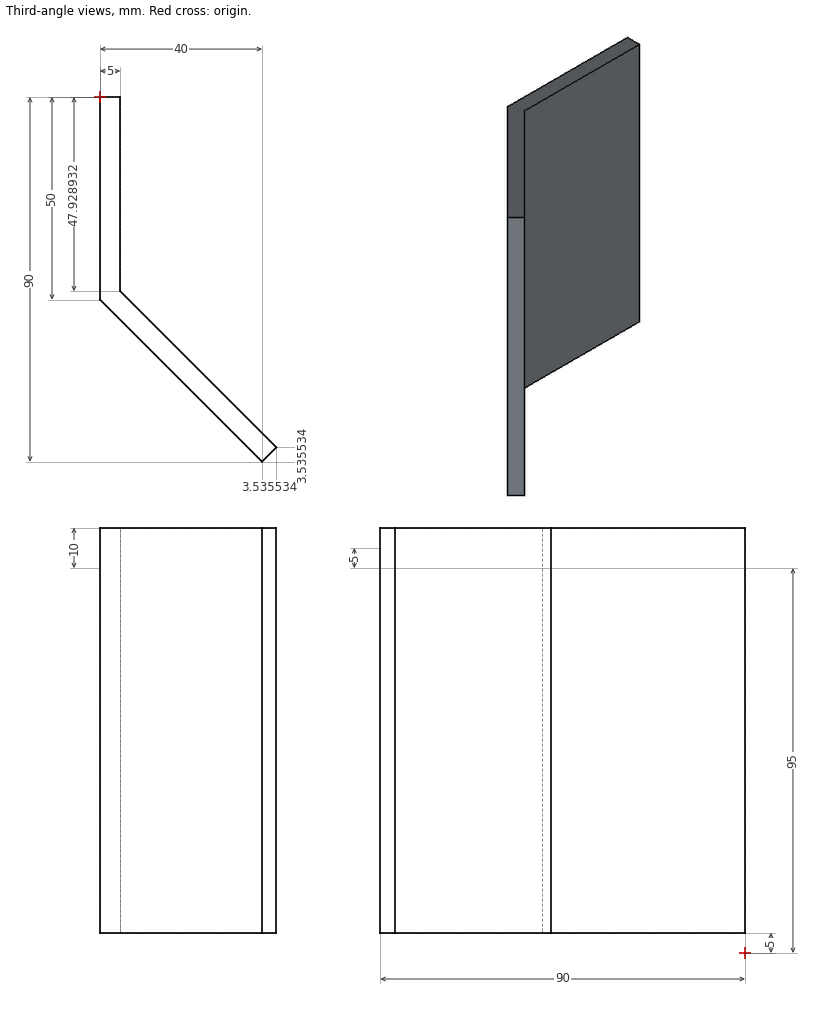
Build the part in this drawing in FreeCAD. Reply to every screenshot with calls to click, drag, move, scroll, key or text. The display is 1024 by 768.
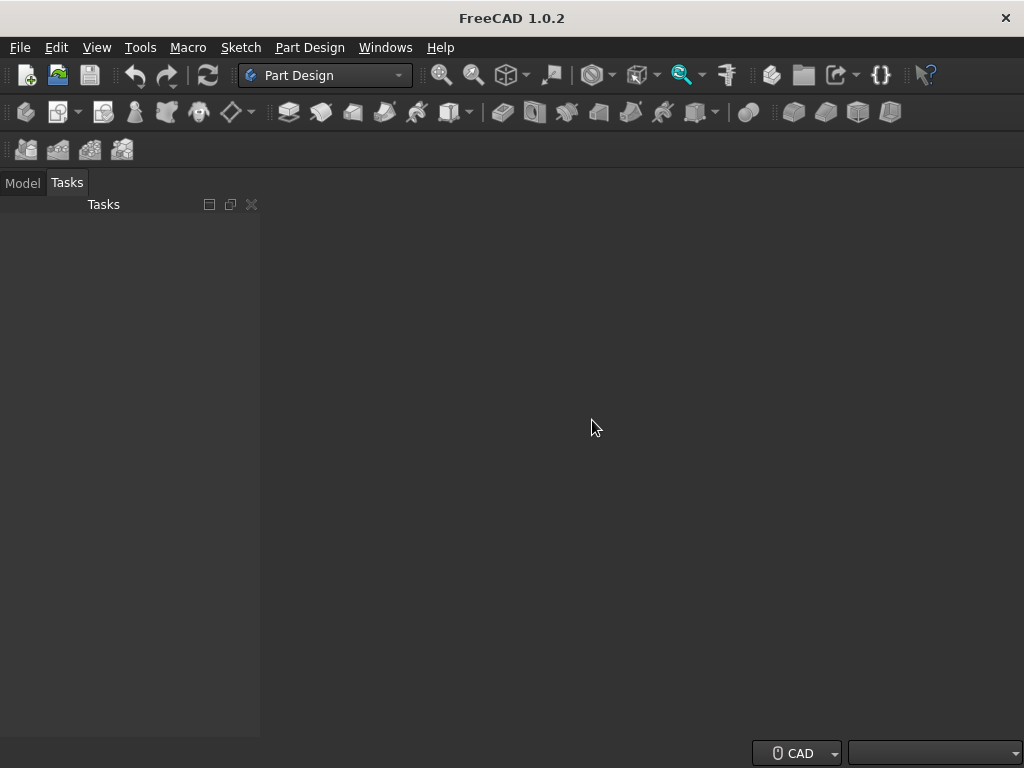
click(26, 76)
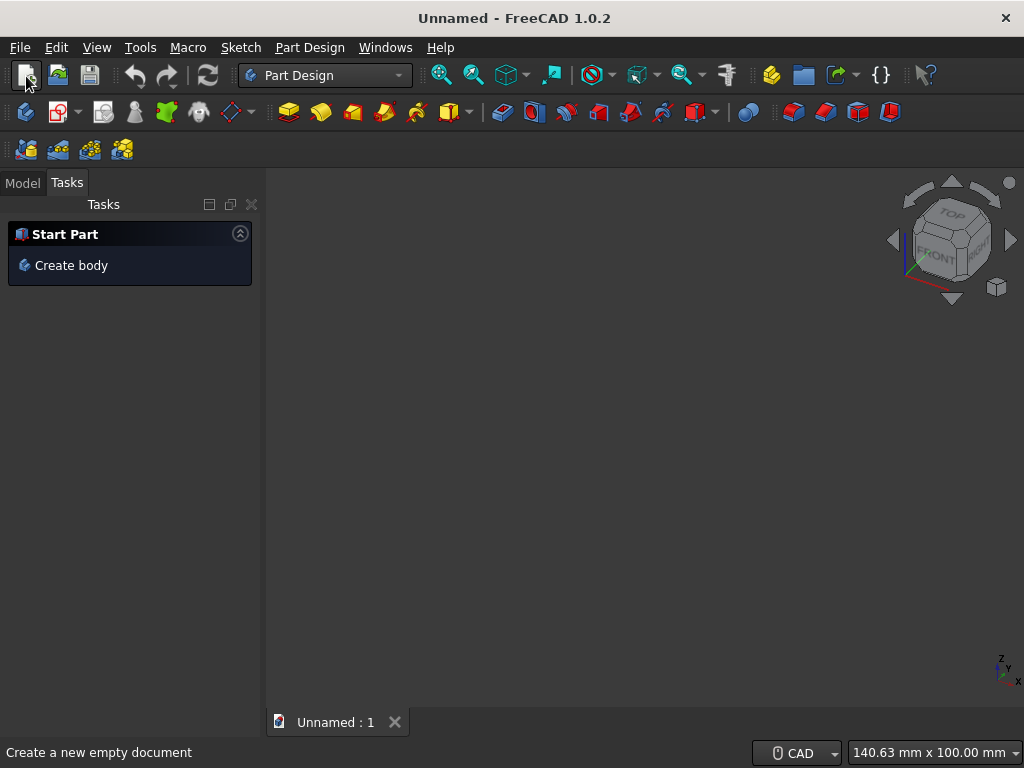
click(58, 112)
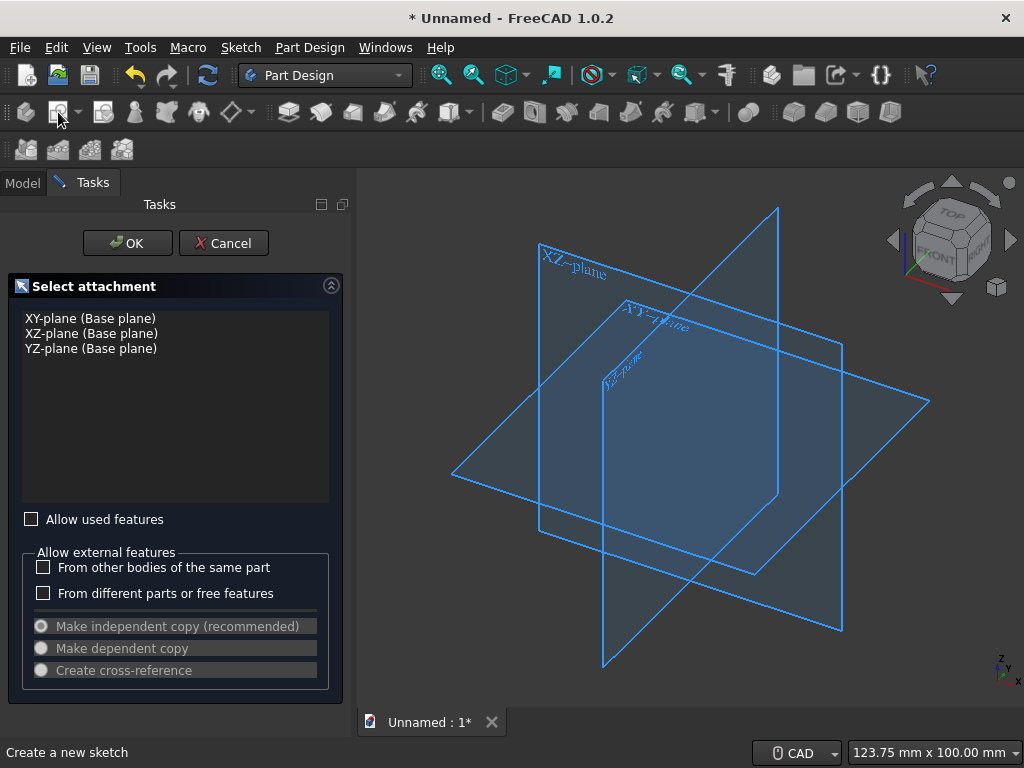
click(82, 318)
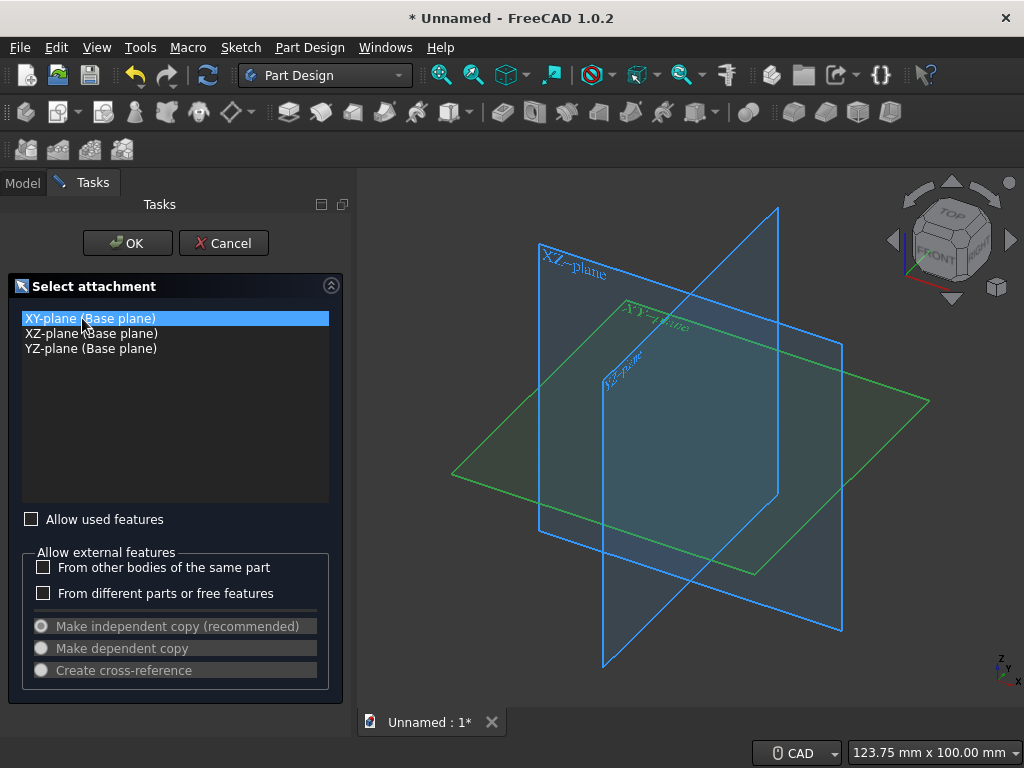
click(128, 243)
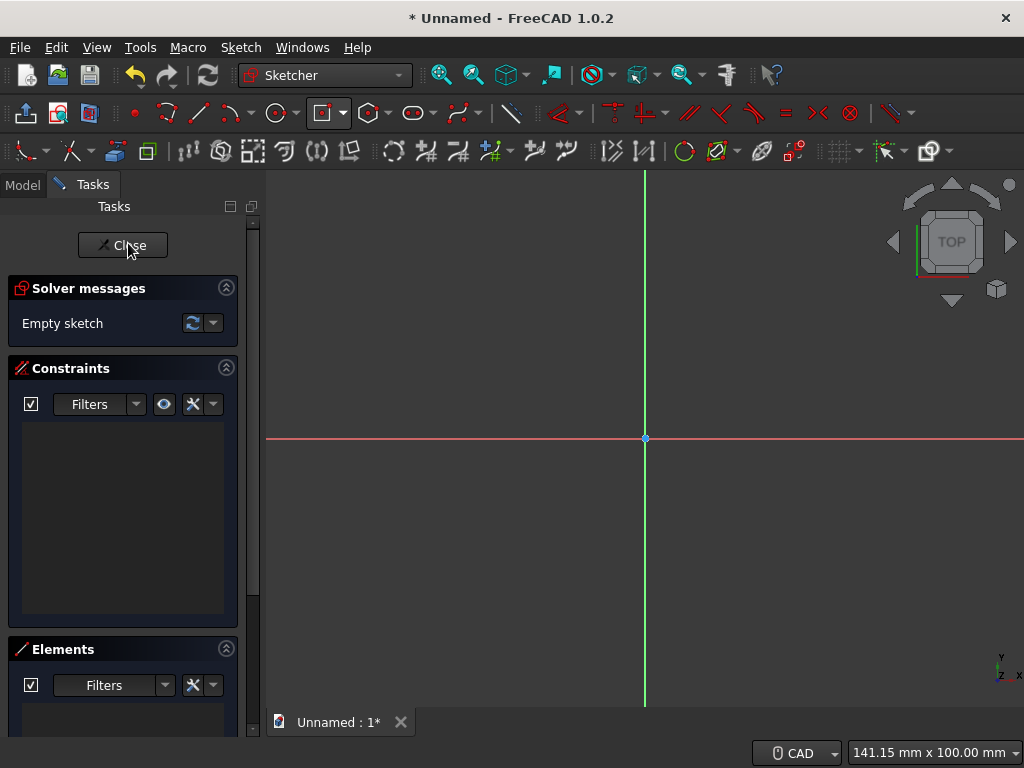
scroll(351, 198, down, 3)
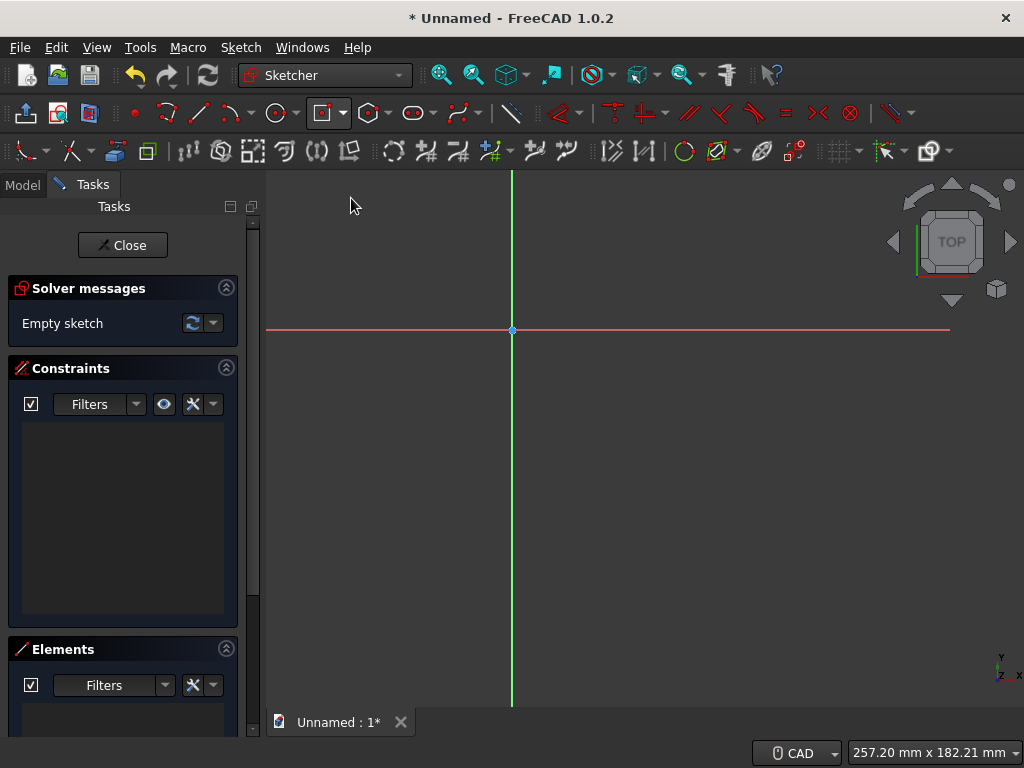
click(168, 114)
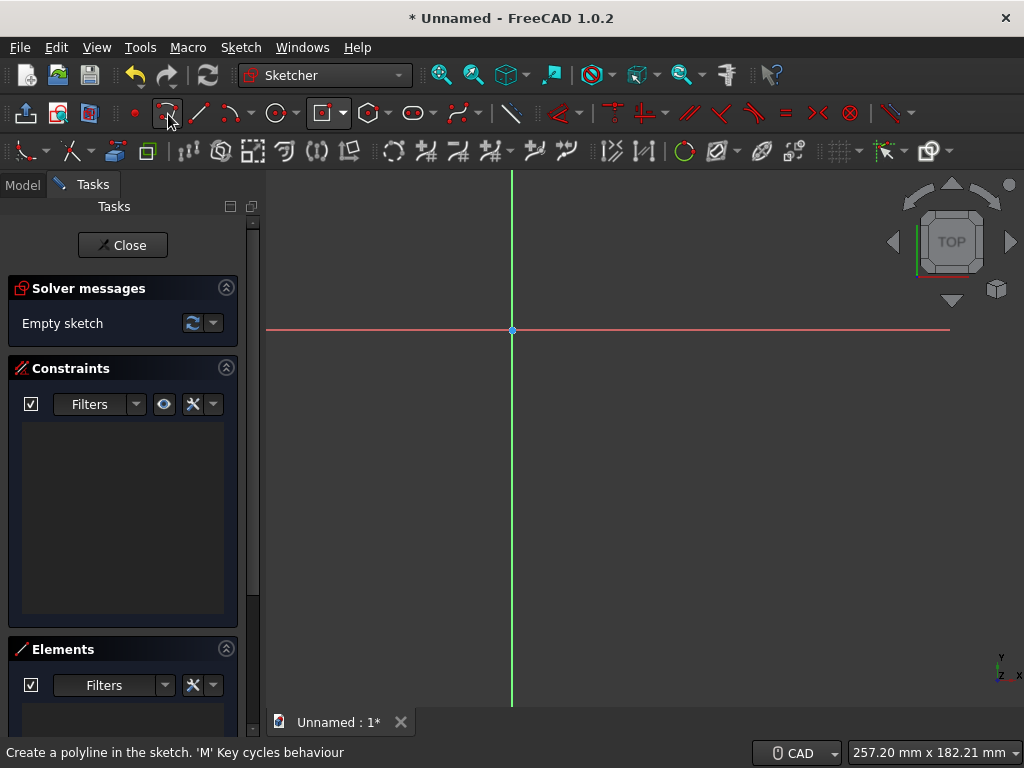
click(512, 330)
click(521, 477)
click(630, 595)
click(641, 585)
click(527, 471)
click(527, 339)
click(512, 330)
key(Escape)
key(Escape)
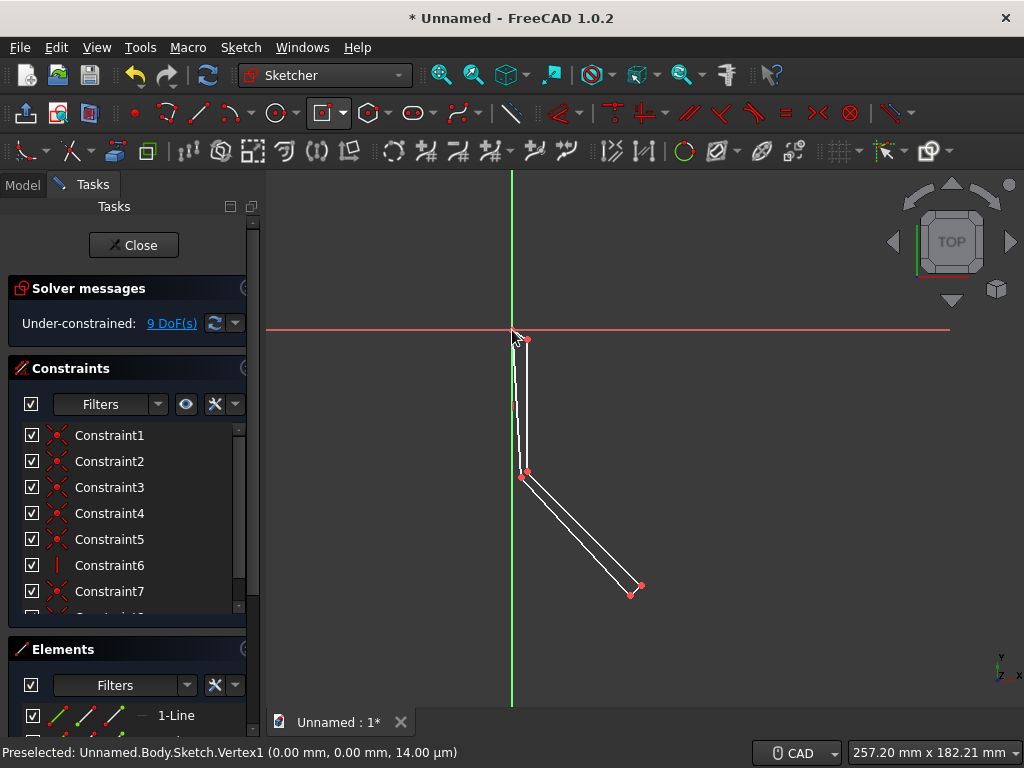
click(515, 374)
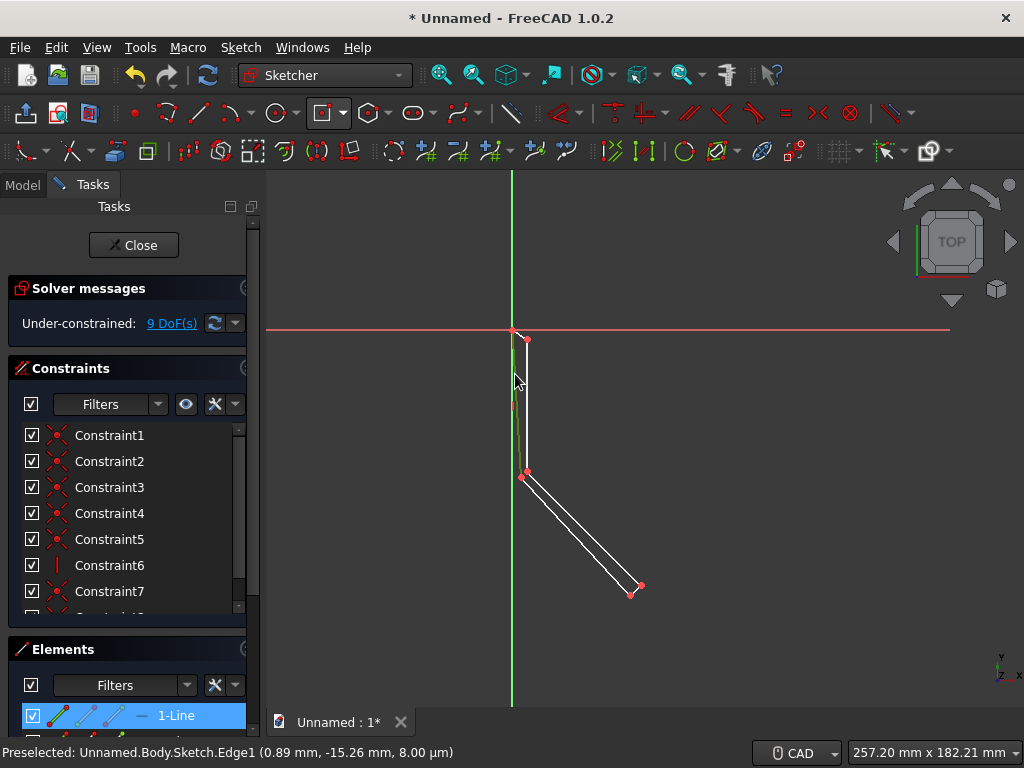
key(v)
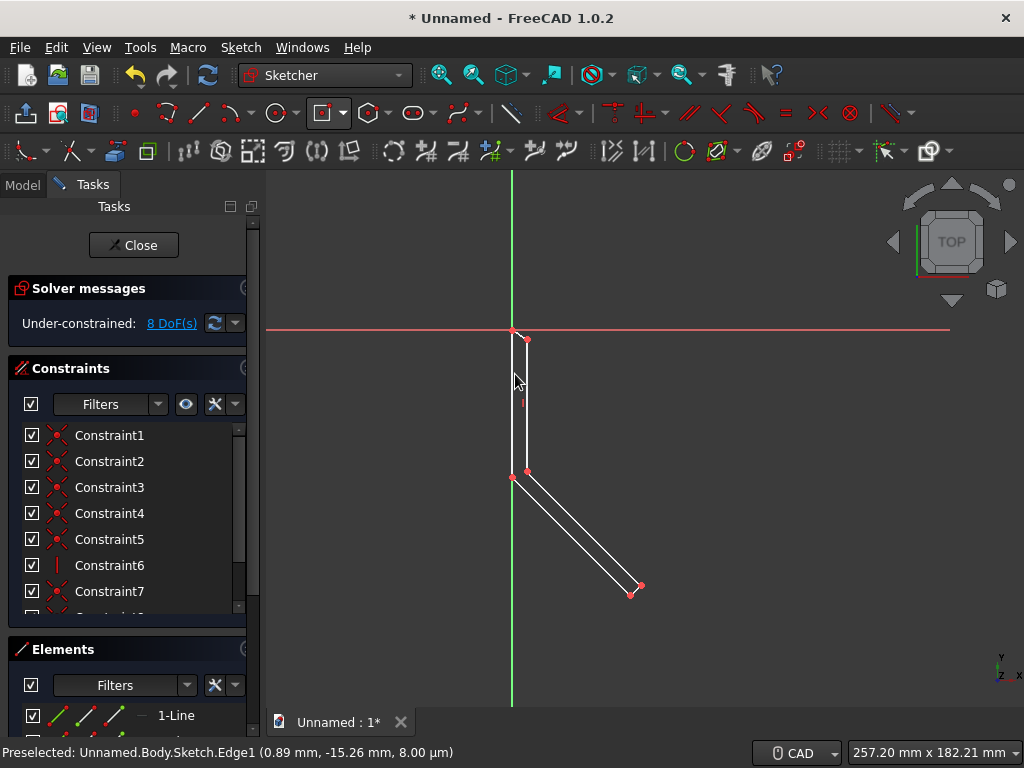
scroll(521, 336, up, 5)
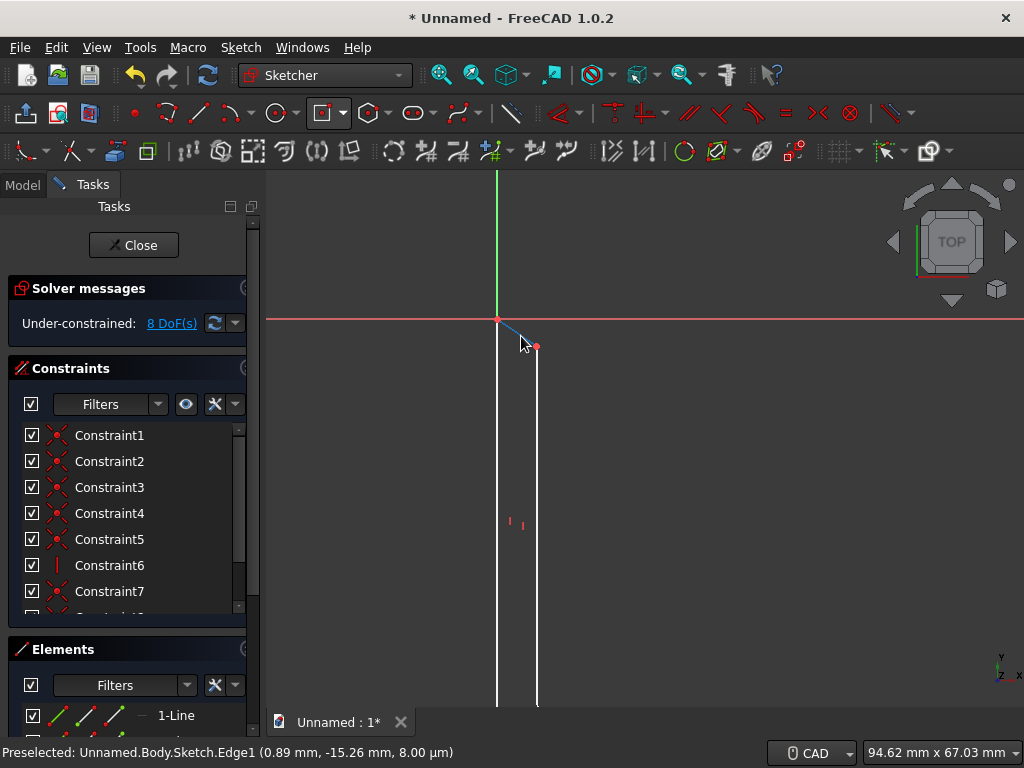
click(521, 335)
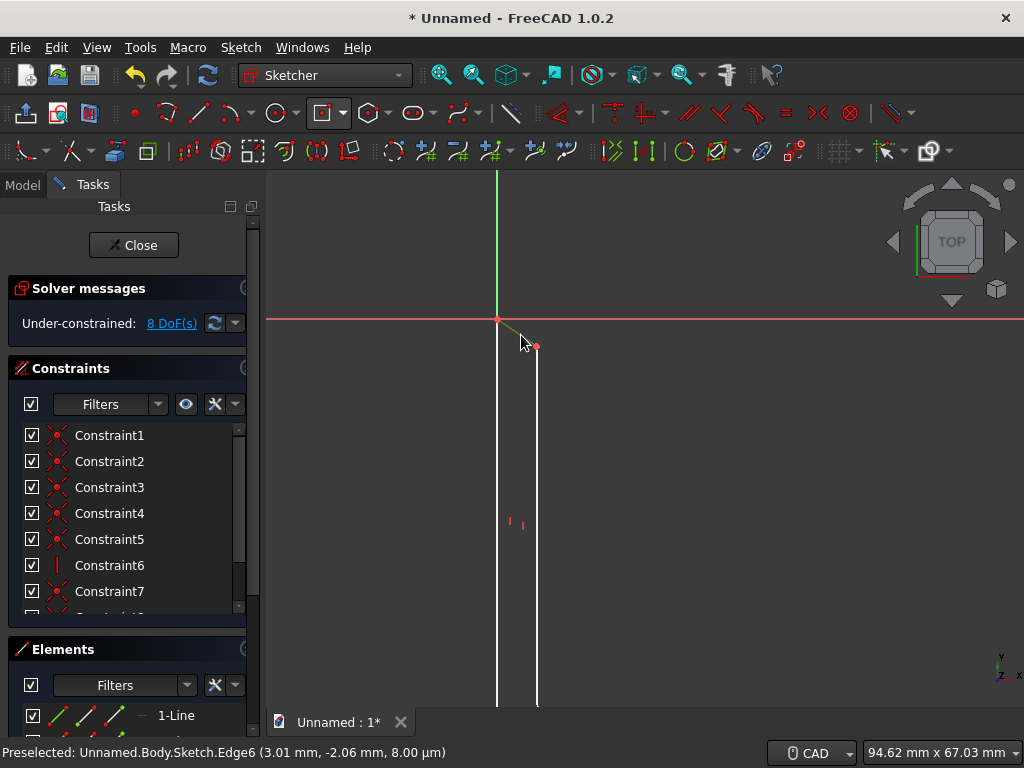
key(h)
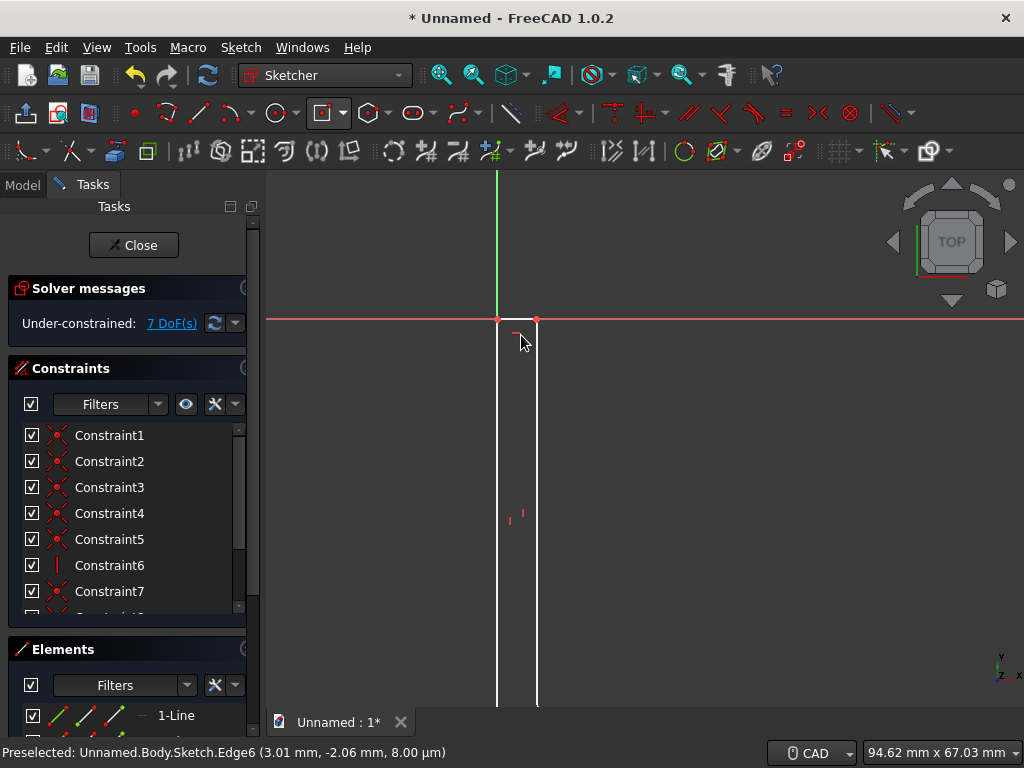
click(558, 114)